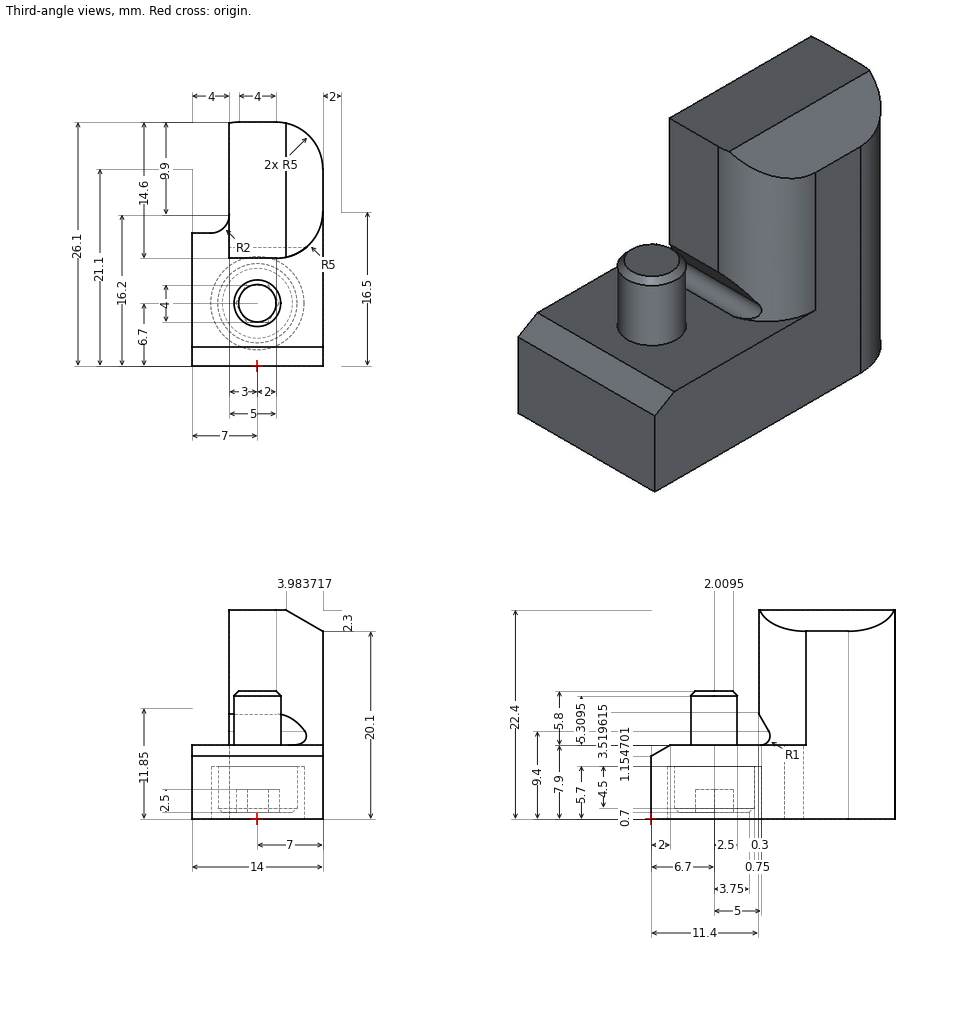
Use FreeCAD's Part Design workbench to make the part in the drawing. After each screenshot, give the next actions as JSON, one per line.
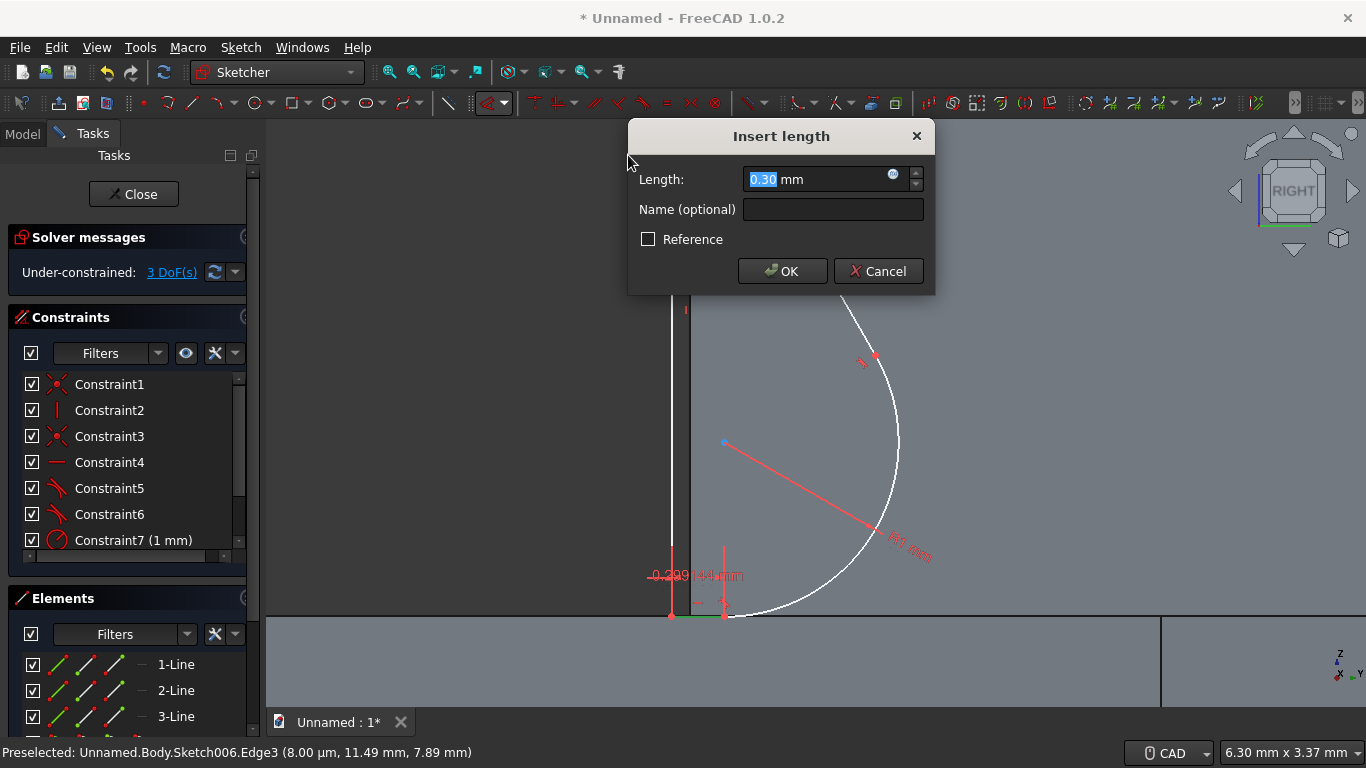
{"action": "type", "text": "0.3"}
{"action": "key", "text": "Return"}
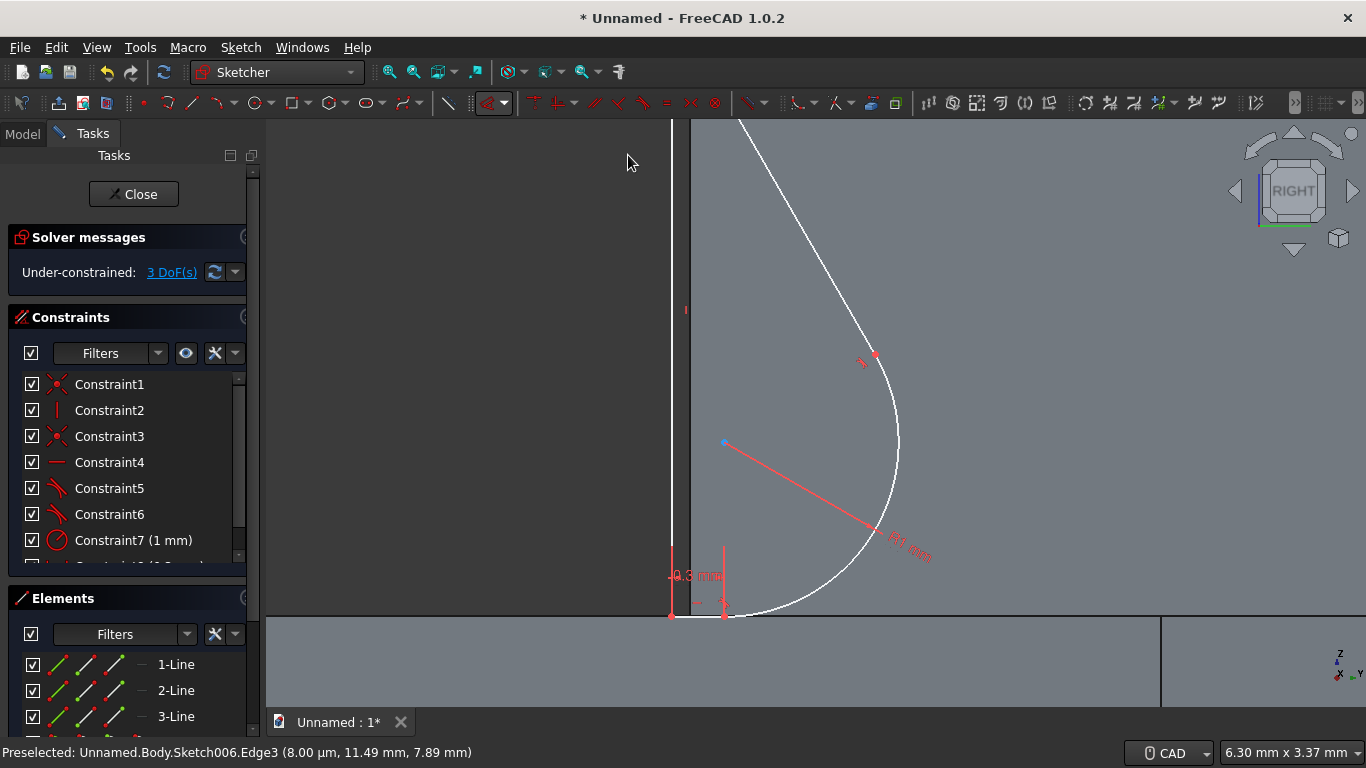
{"action": "left_click", "coordinate": [875, 355]}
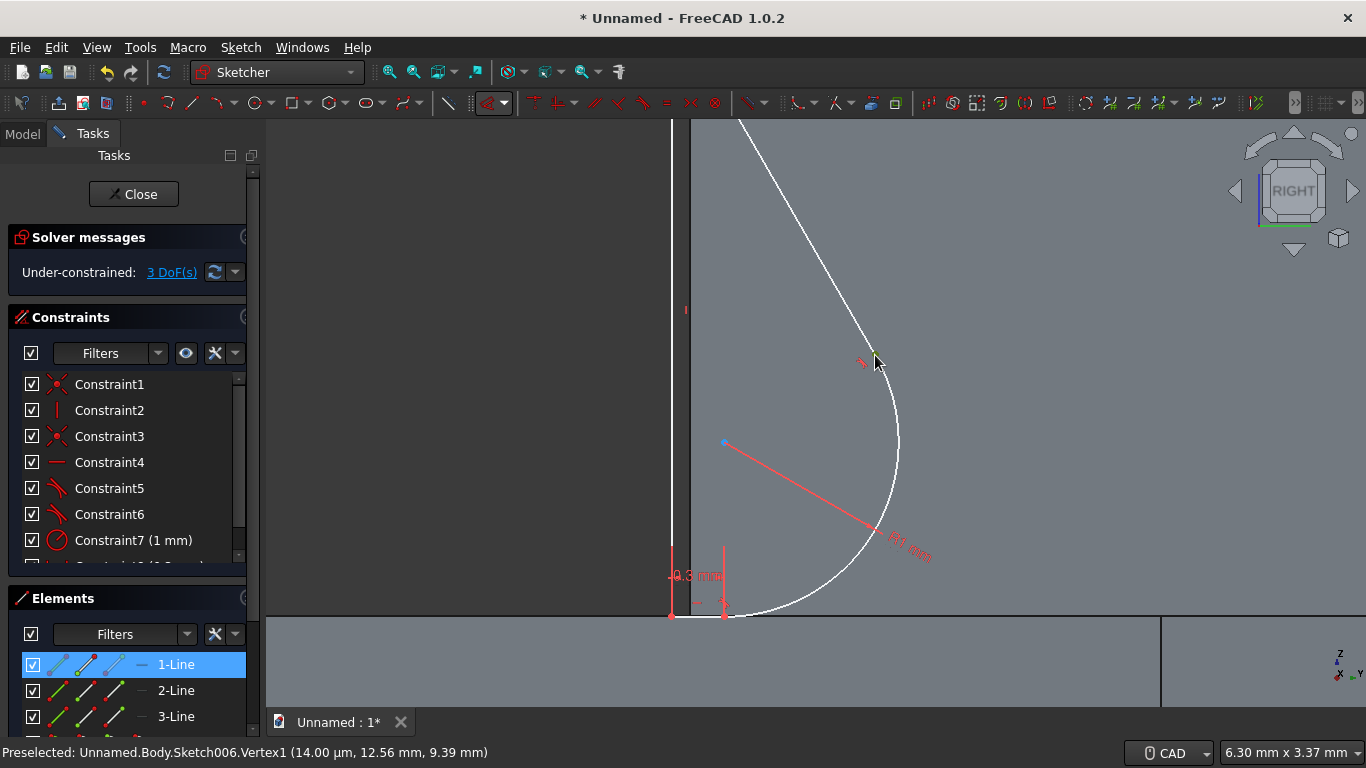
{"action": "key", "text": "i"}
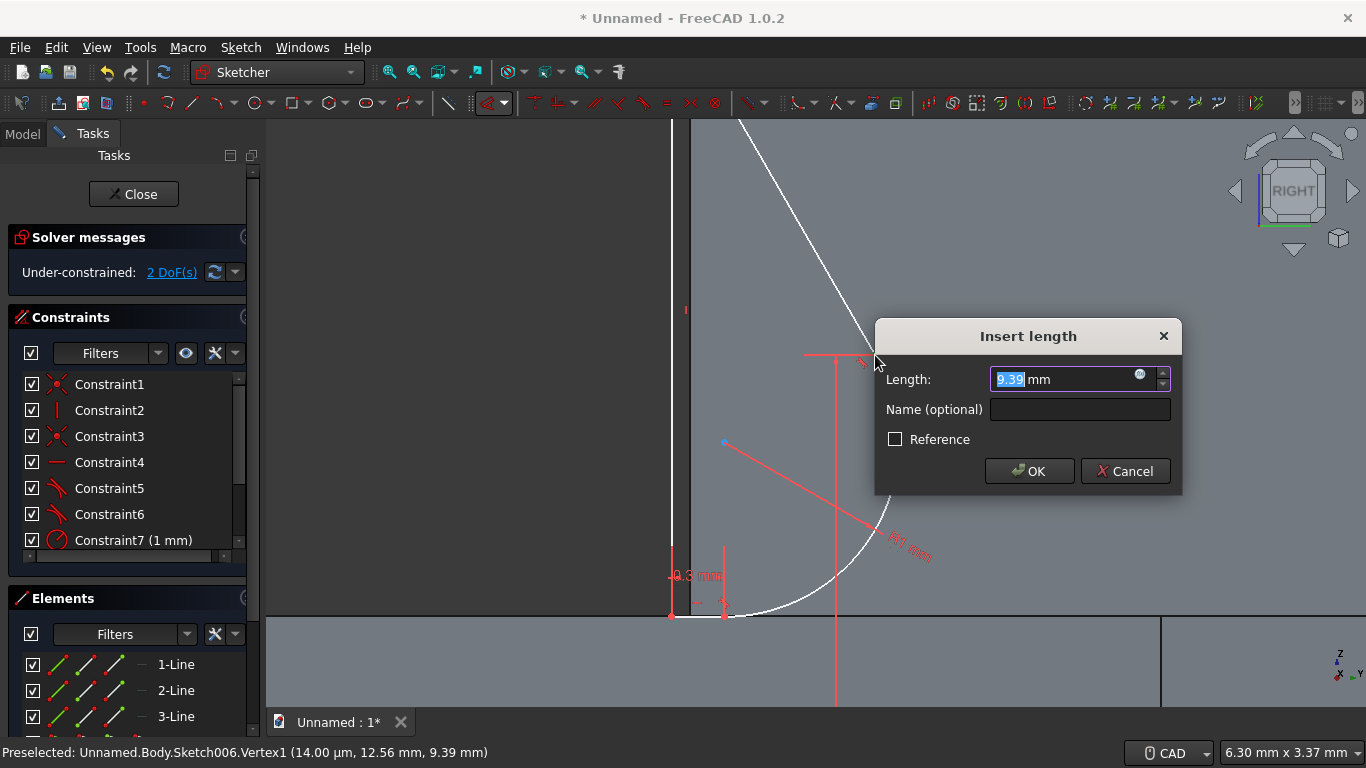
{"action": "type", "text": "9.4"}
{"action": "key", "text": "Return"}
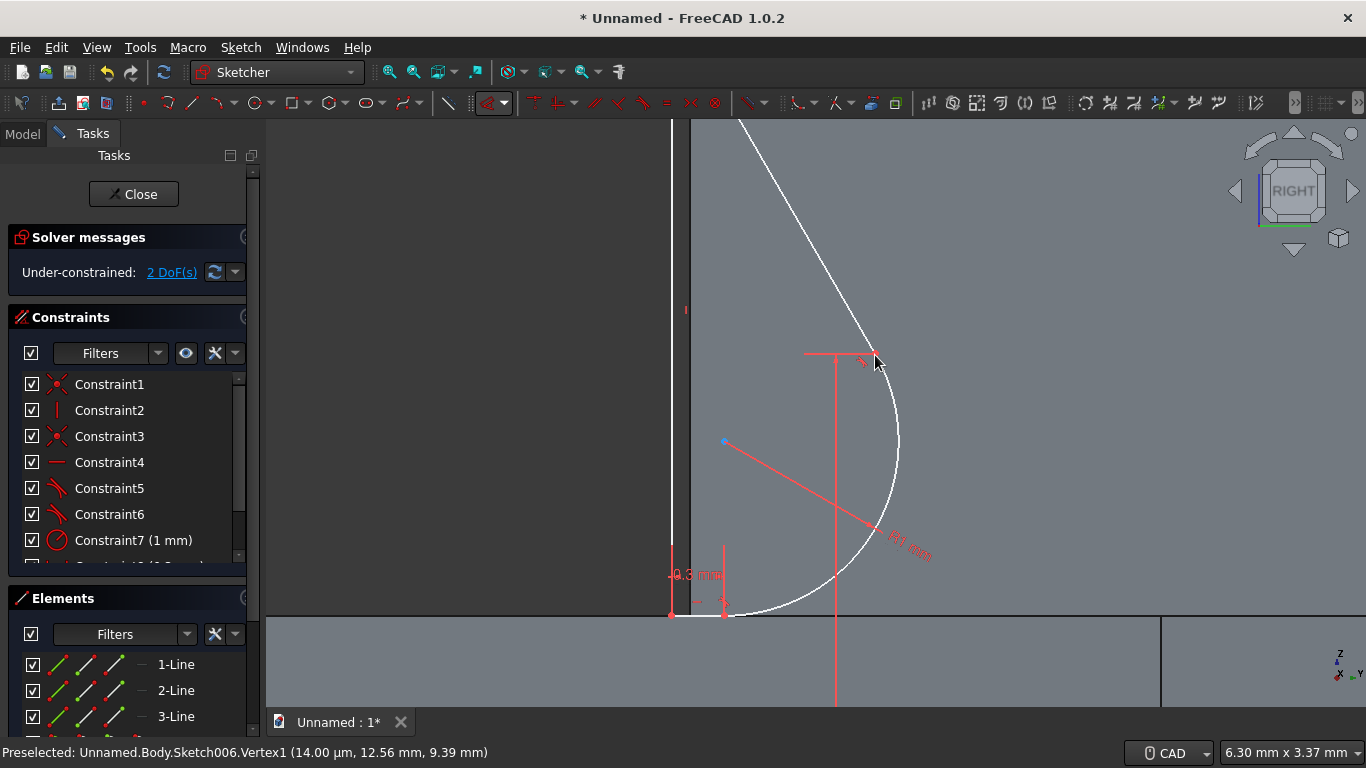
{"action": "scroll", "coordinate": [693, 626], "scroll_direction": "down", "scroll_amount": 2}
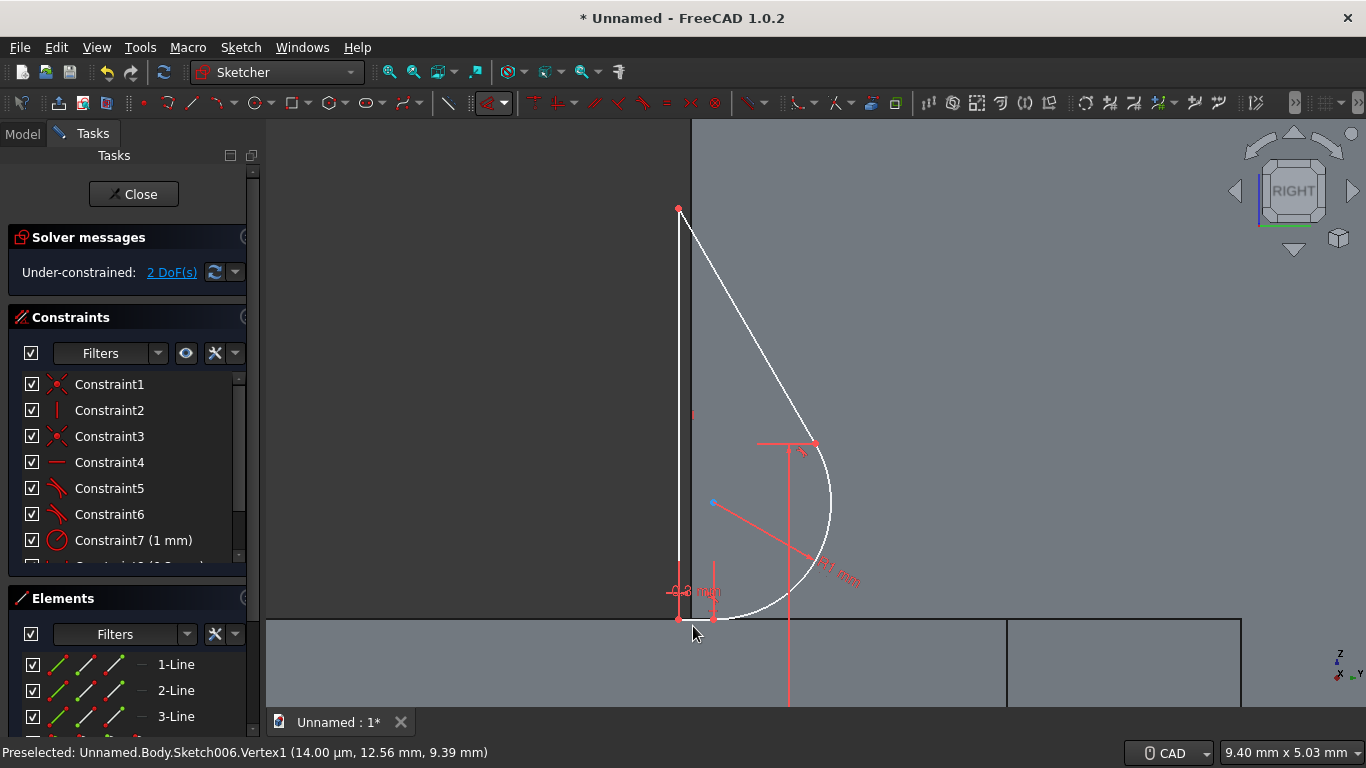
{"action": "left_click", "coordinate": [679, 209]}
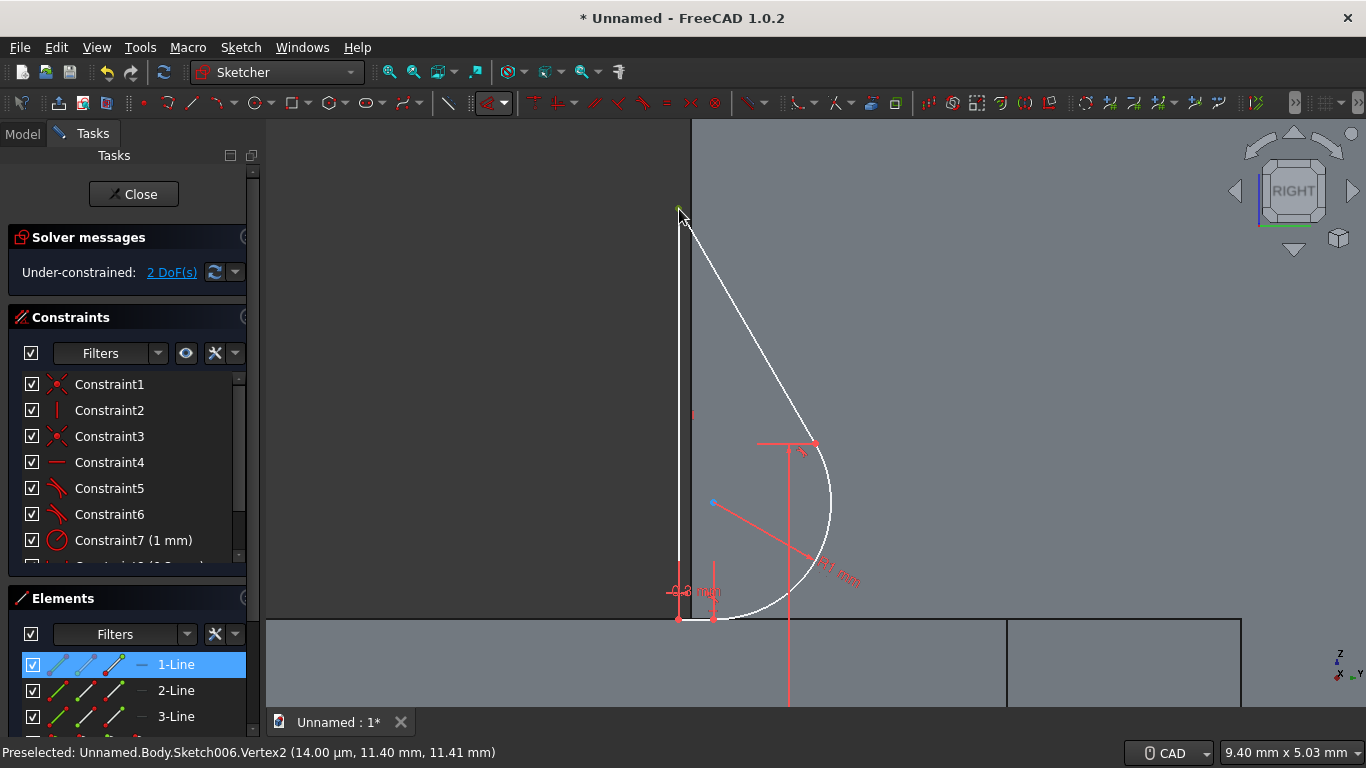
{"action": "left_click", "coordinate": [506, 104]}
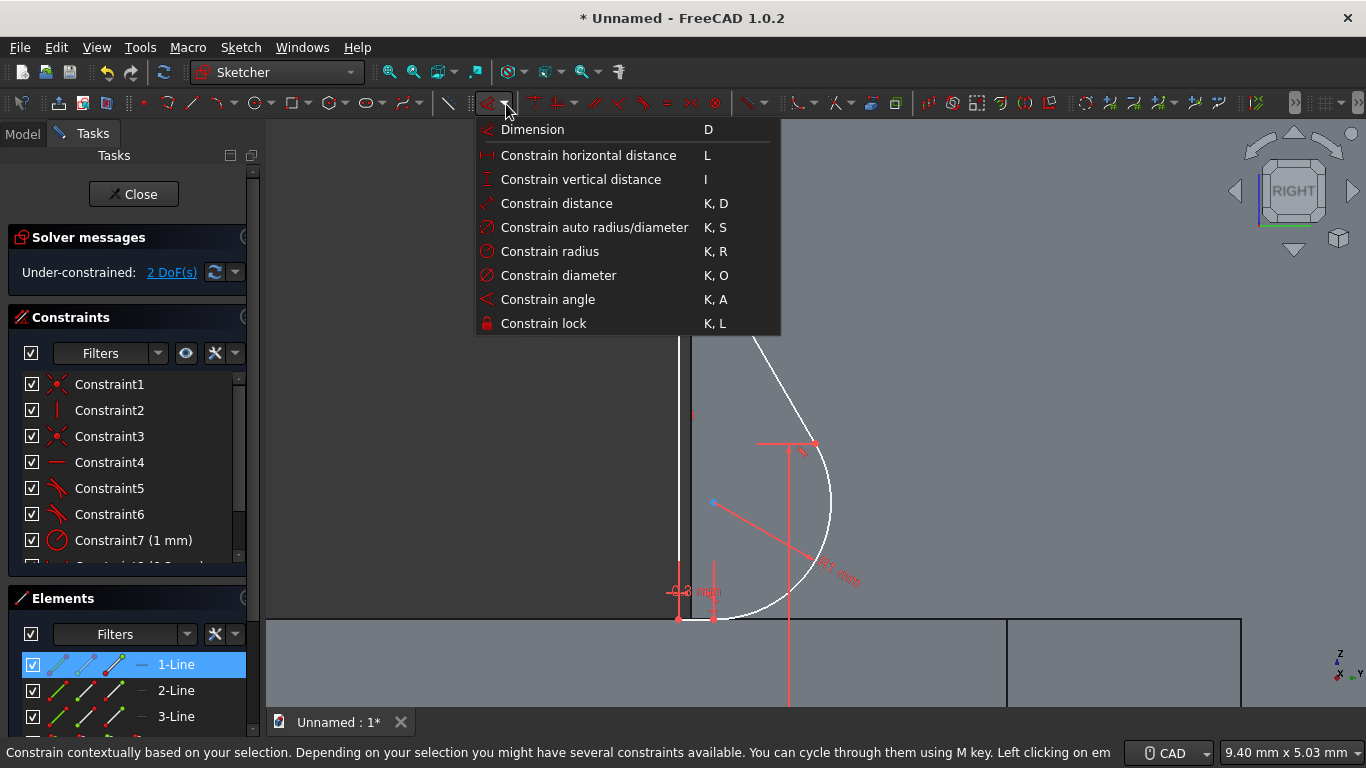
{"action": "left_click", "coordinate": [628, 155]}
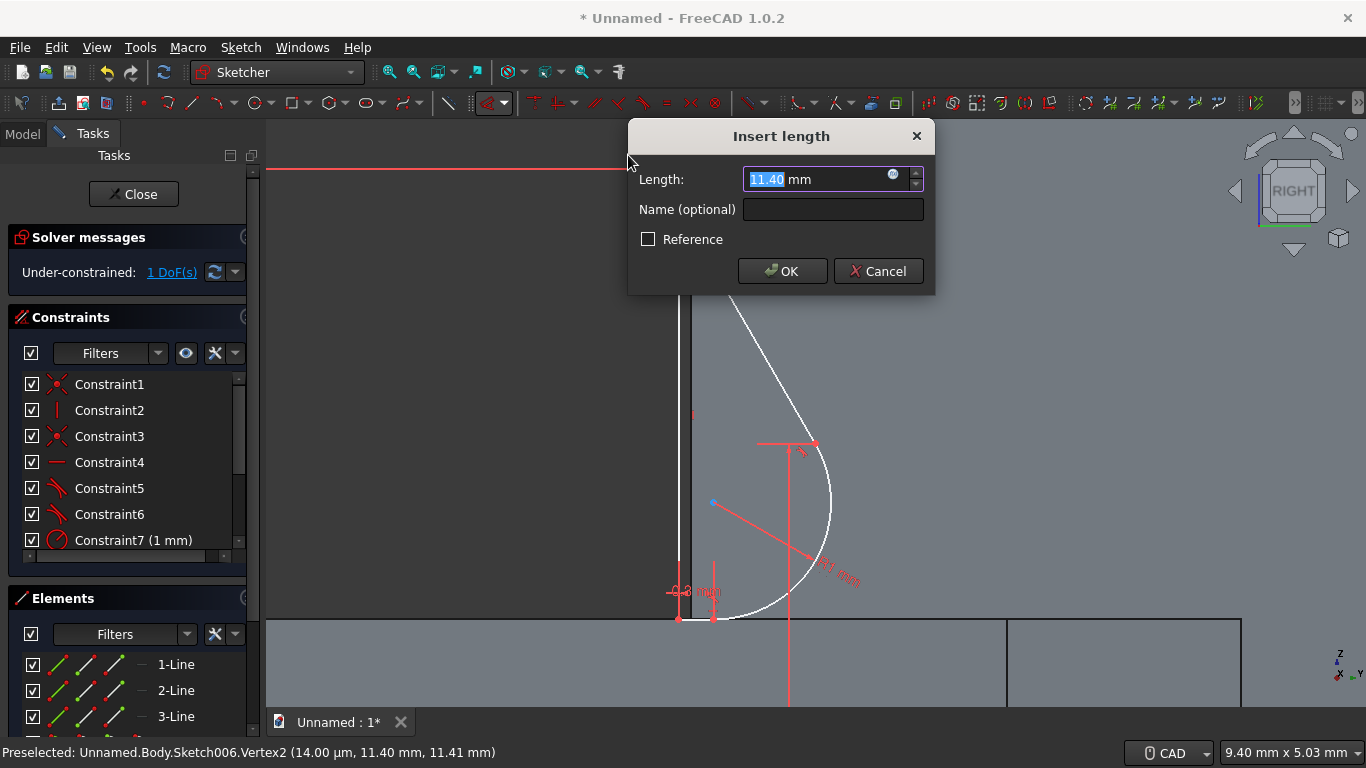
{"action": "type", "text": "11.4"}
{"action": "key", "text": "Return"}